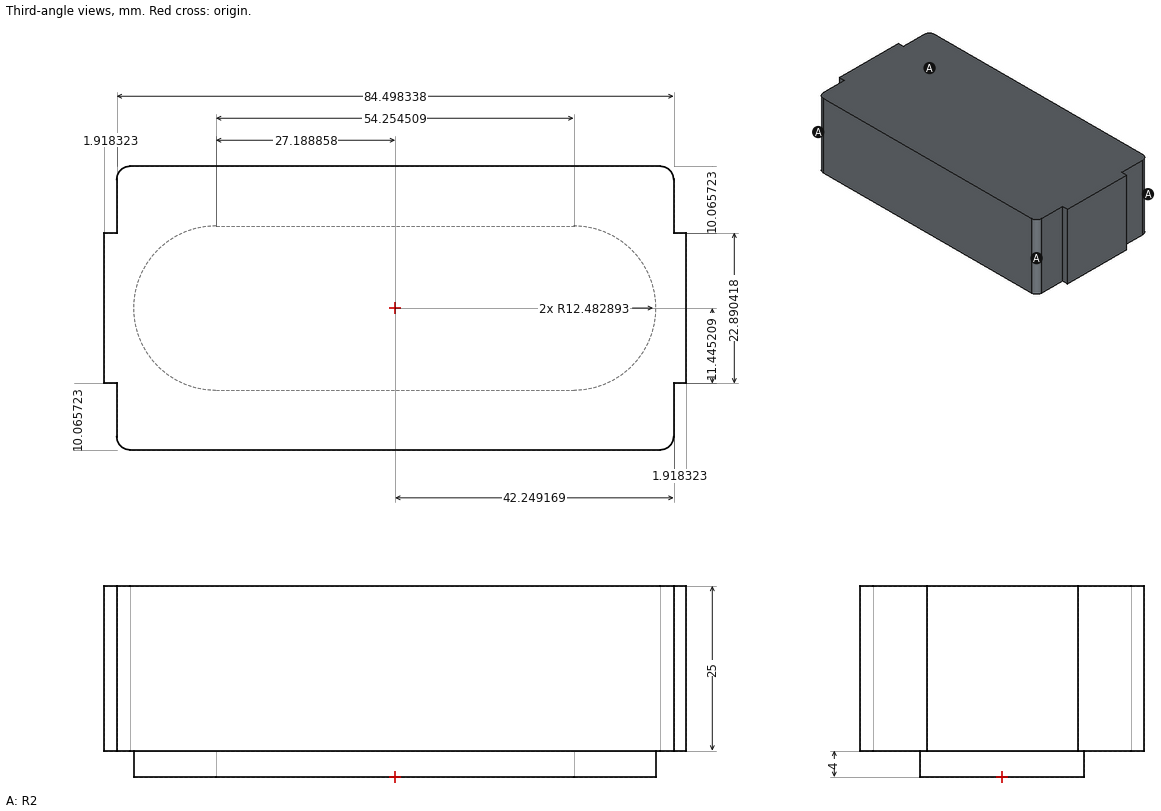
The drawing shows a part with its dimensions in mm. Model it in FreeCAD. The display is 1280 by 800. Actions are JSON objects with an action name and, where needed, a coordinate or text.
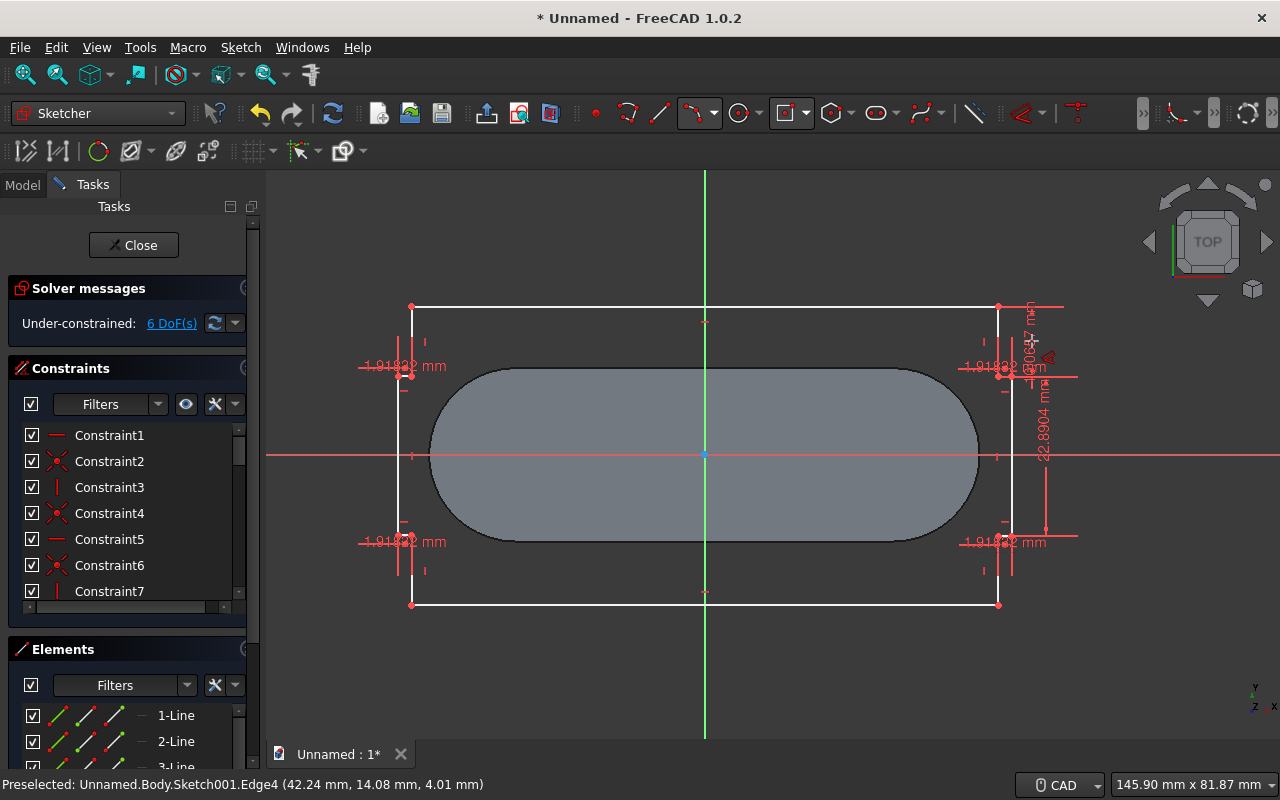
{"action": "left_click", "coordinate": [822, 307]}
{"action": "left_click", "coordinate": [570, 273]}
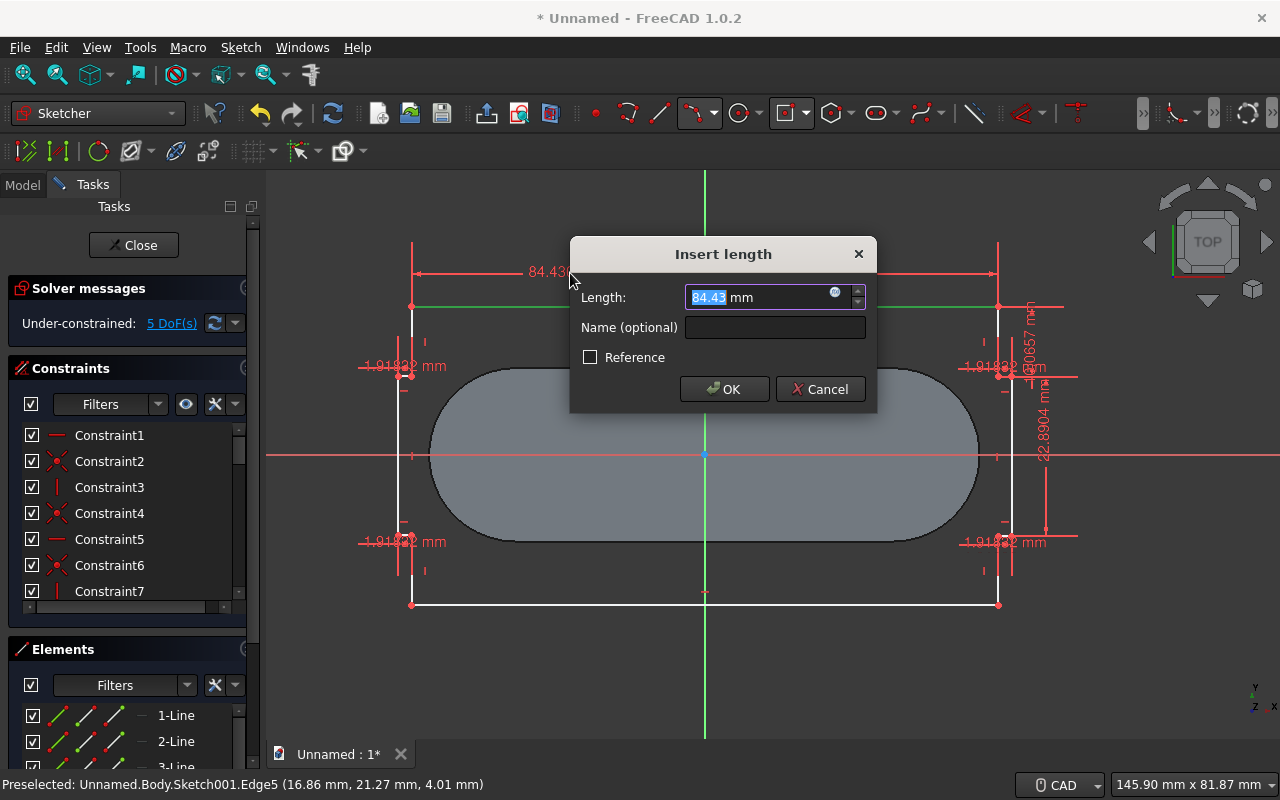
{"action": "type", "text": "84.498338"}
{"action": "key", "text": "Return"}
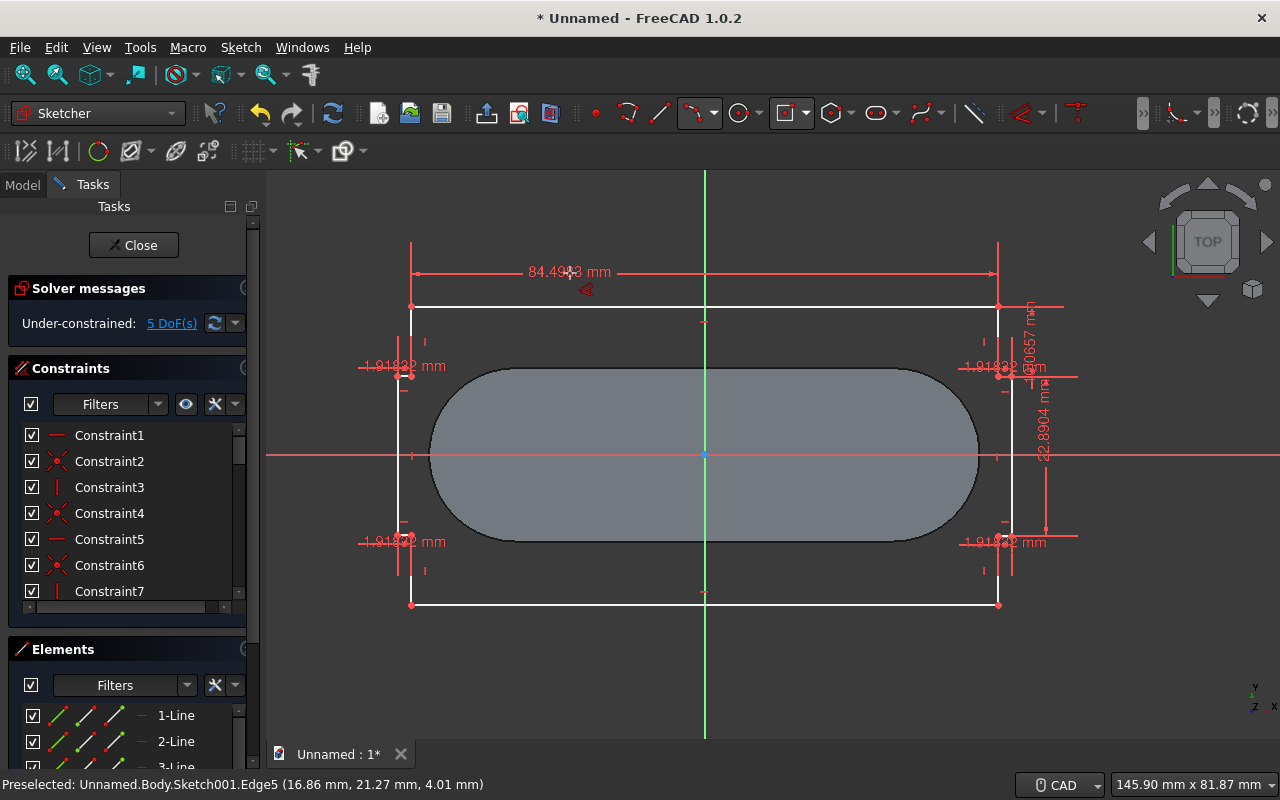
{"action": "left_click", "coordinate": [411, 328]}
{"action": "left_click", "coordinate": [377, 342]}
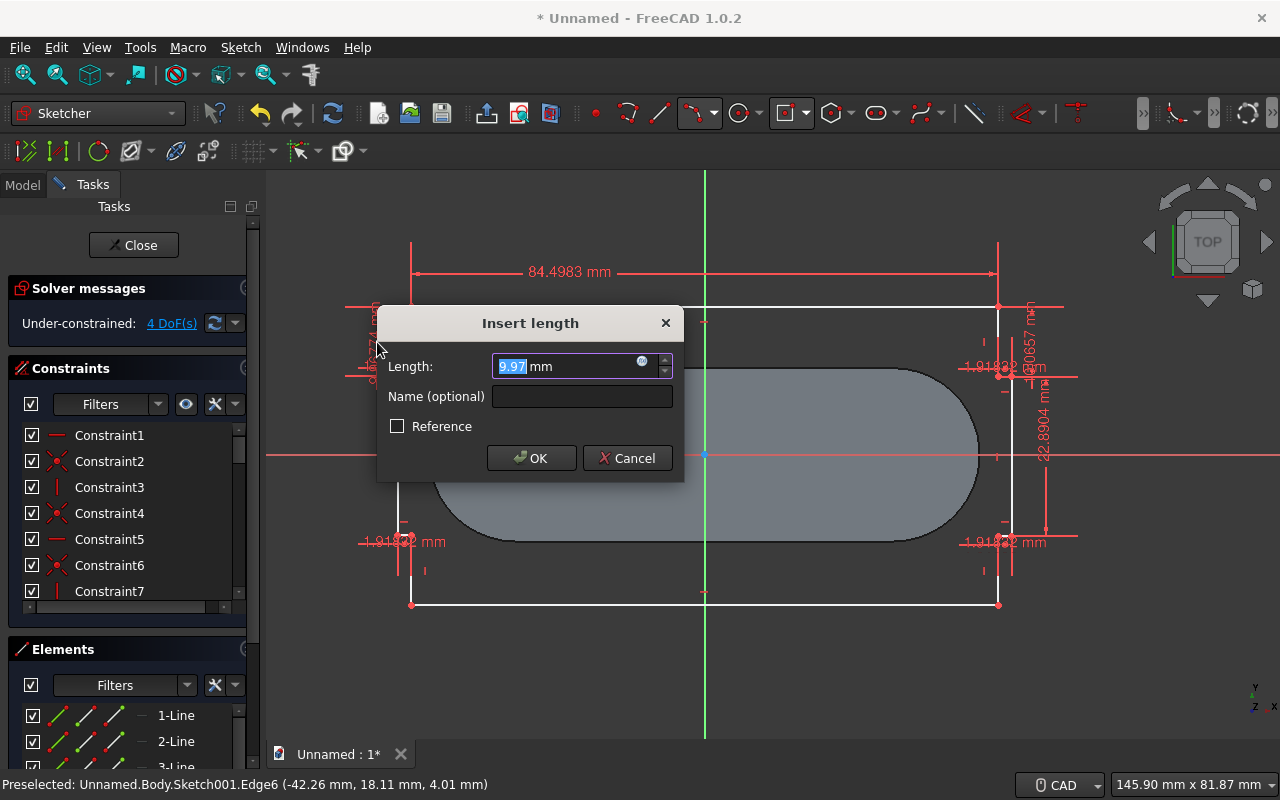
{"action": "type", "text": "10.065723"}
{"action": "key", "text": "Return"}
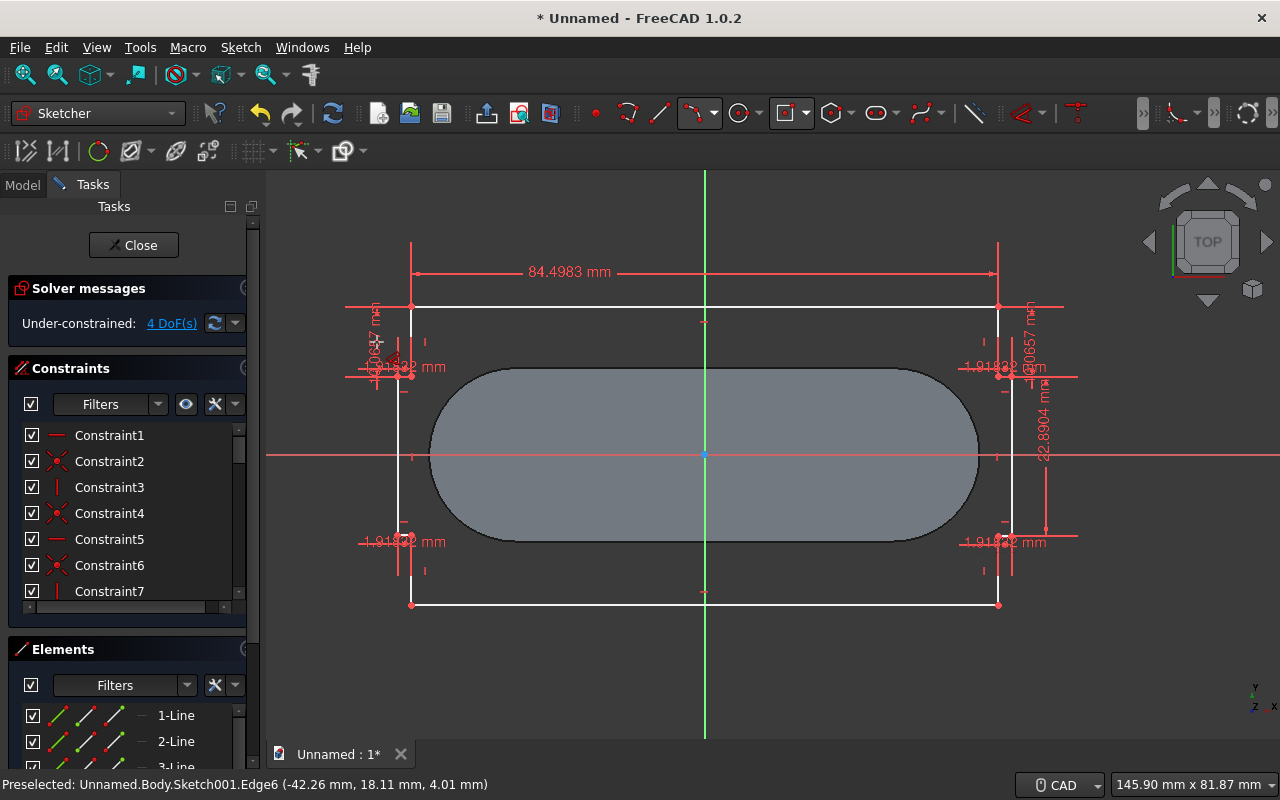
{"action": "left_click", "coordinate": [398, 424]}
{"action": "left_click", "coordinate": [364, 420]}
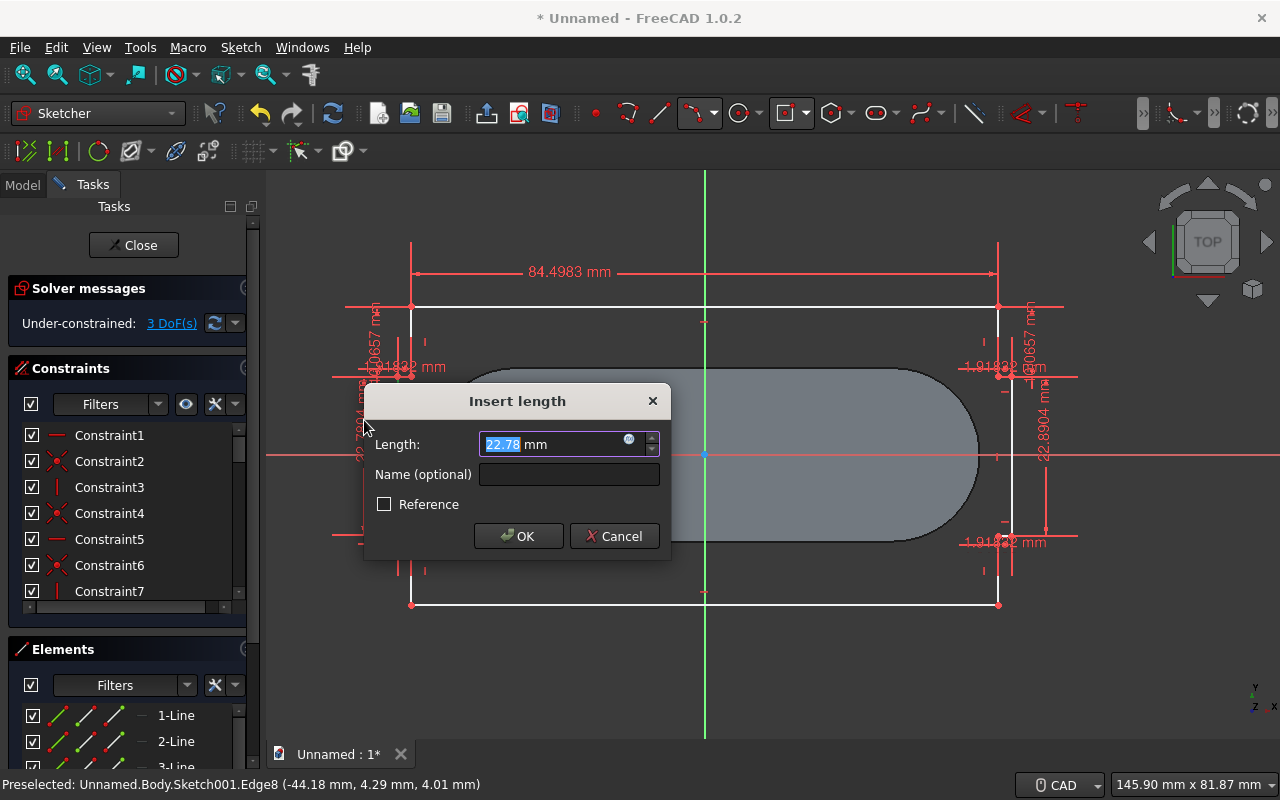
{"action": "type", "text": "22.890418"}
{"action": "key", "text": "Return"}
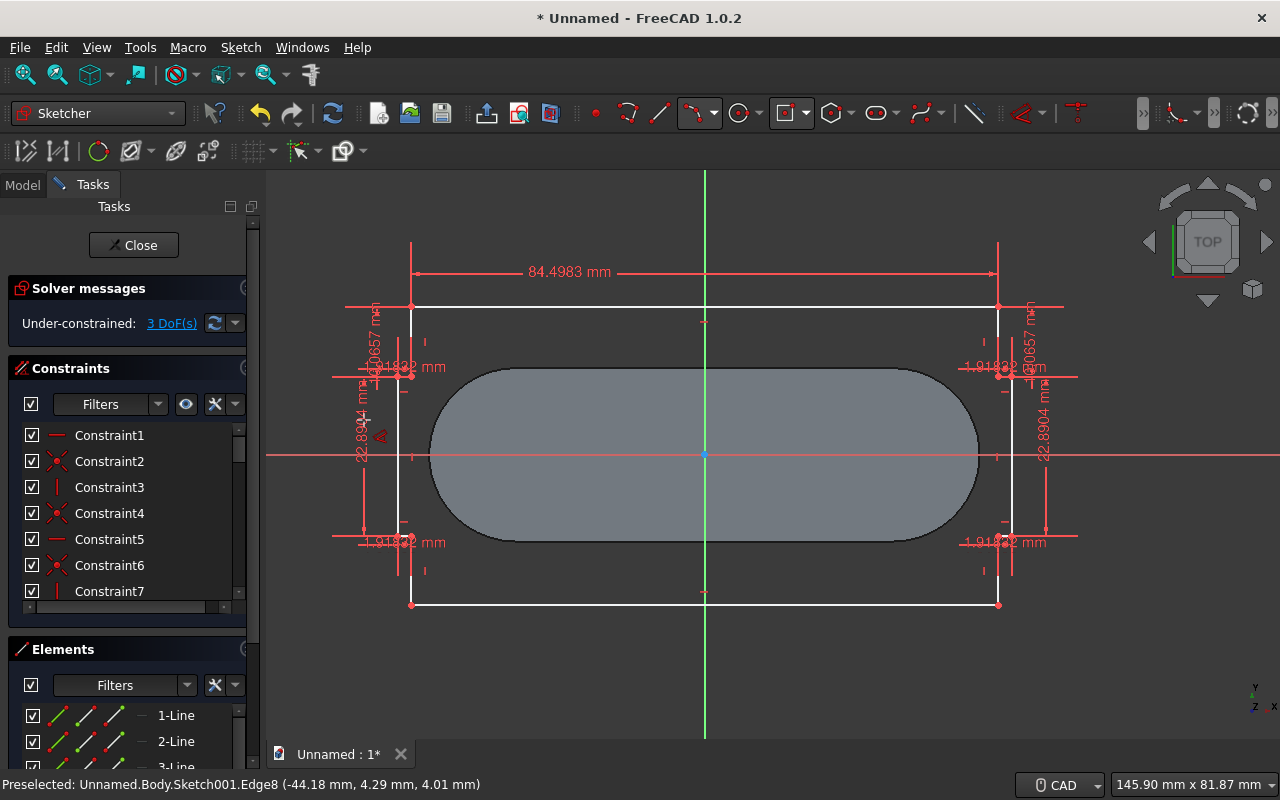
{"action": "left_click", "coordinate": [411, 557]}
{"action": "left_click", "coordinate": [377, 571]}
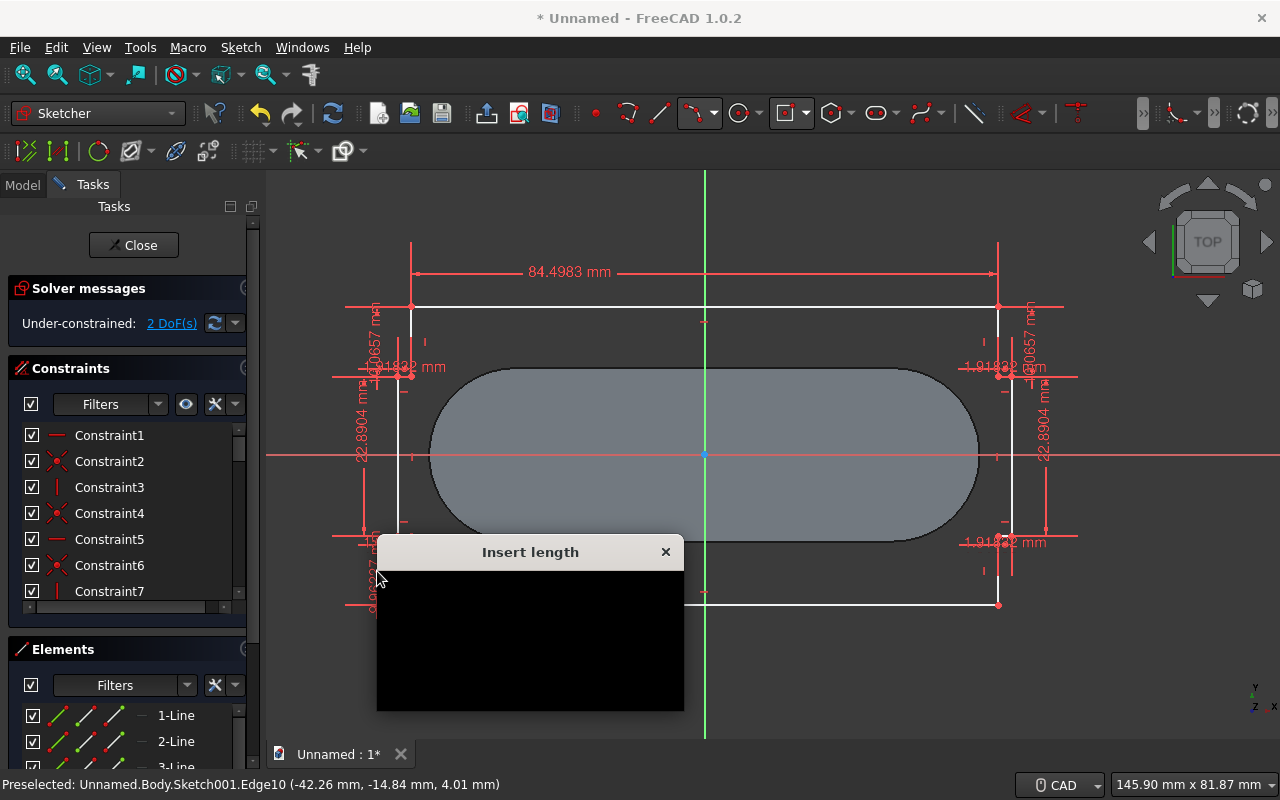
{"action": "type", "text": "10.065723"}
{"action": "key", "text": "Return"}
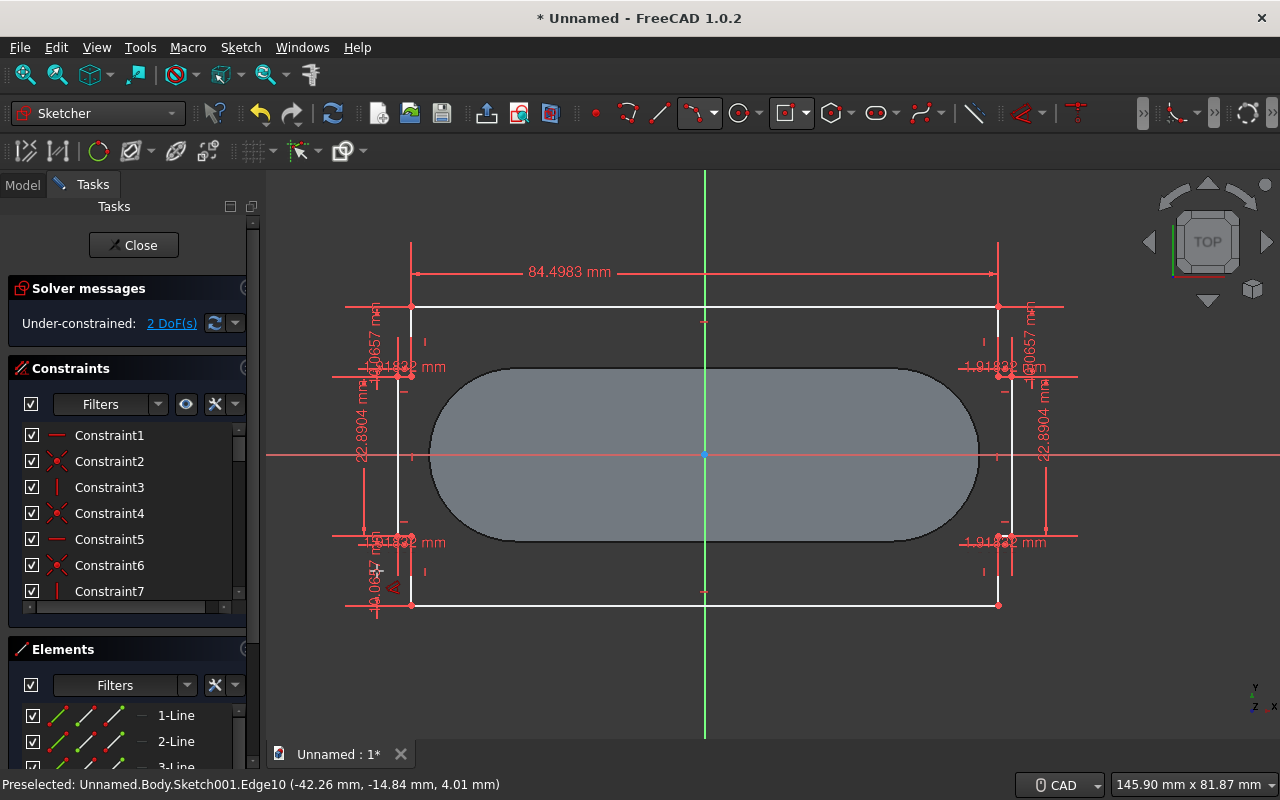
{"action": "left_click", "coordinate": [998, 536]}
{"action": "left_click", "coordinate": [852, 570]}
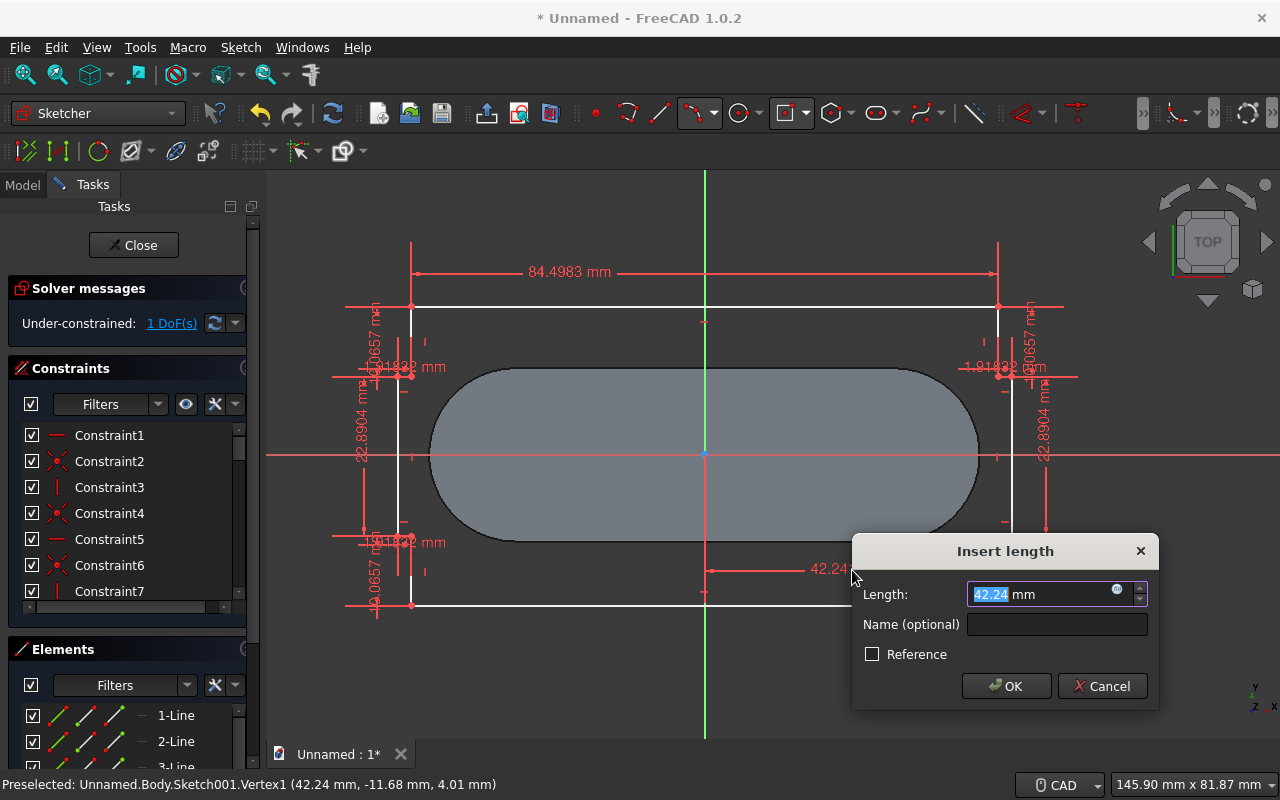
{"action": "type", "text": "42.249169"}
{"action": "key", "text": "Return"}